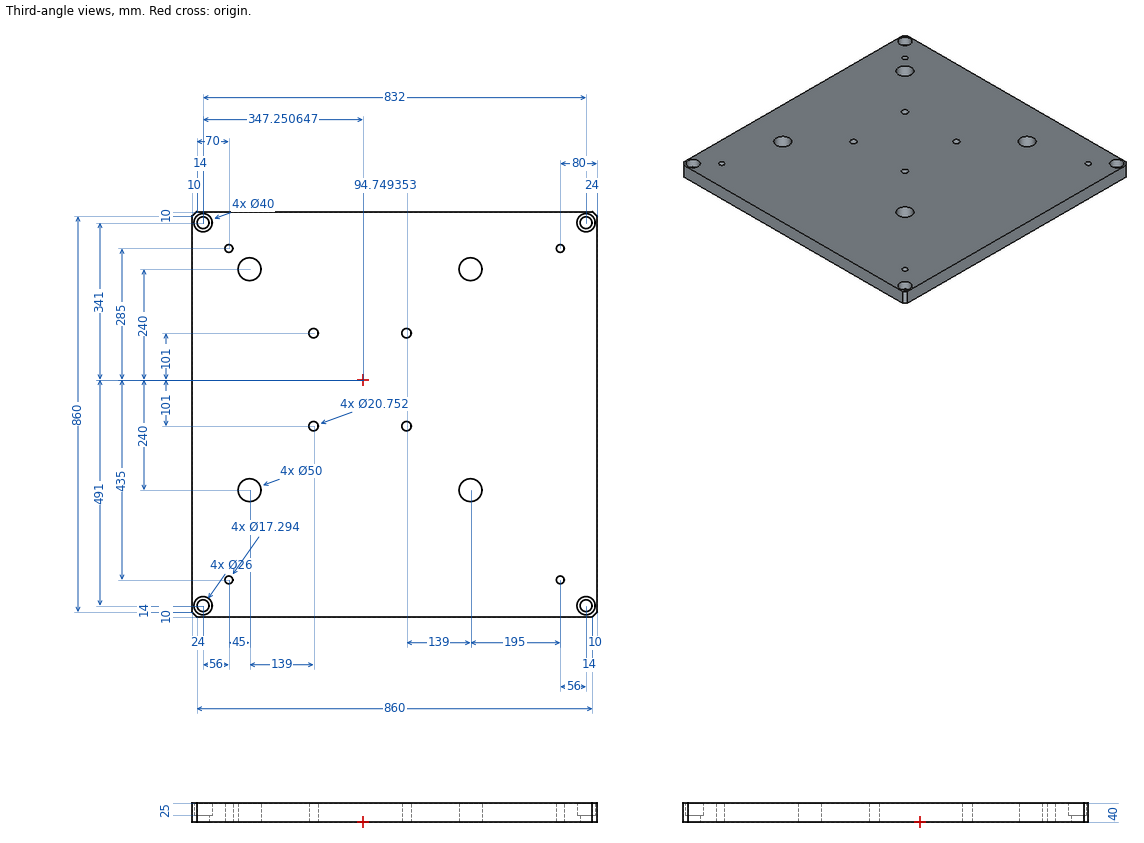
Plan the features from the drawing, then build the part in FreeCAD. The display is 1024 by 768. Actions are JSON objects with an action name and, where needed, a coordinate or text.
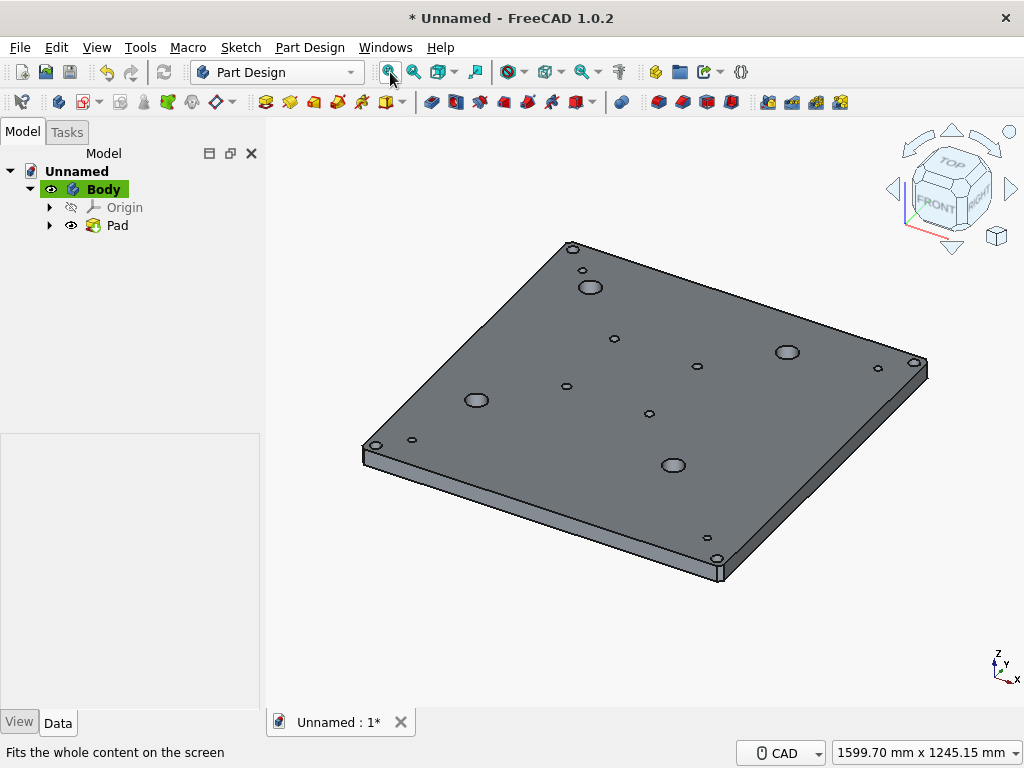
{"action": "left_click", "coordinate": [778, 408]}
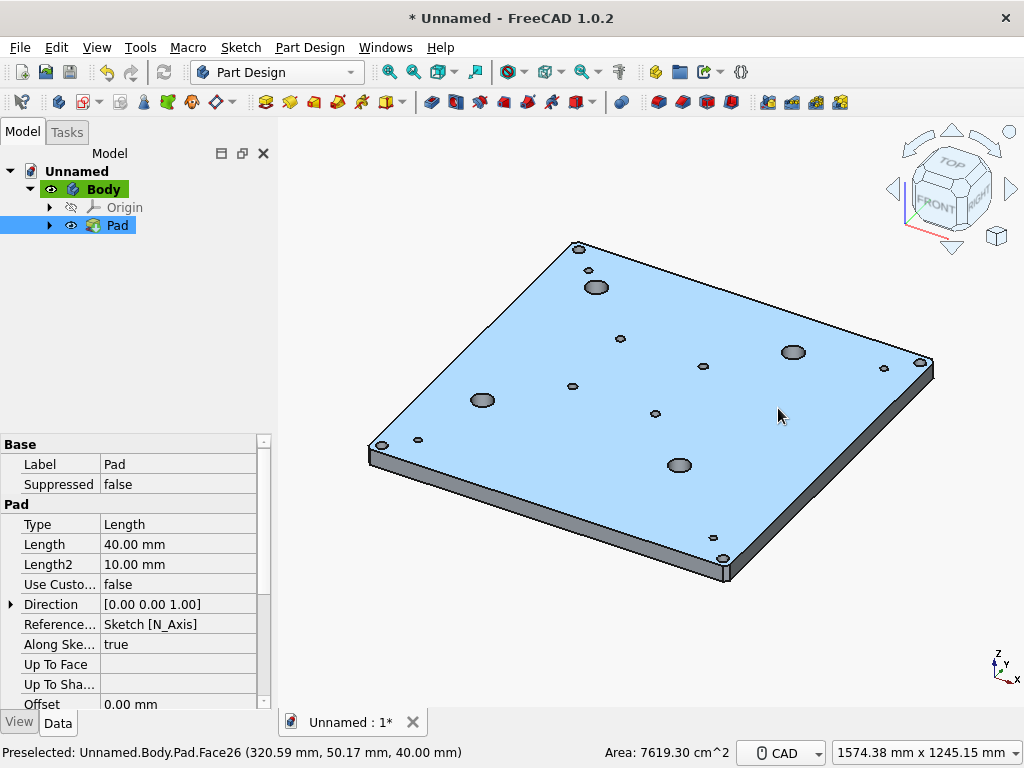
{"action": "left_click", "coordinate": [84, 102]}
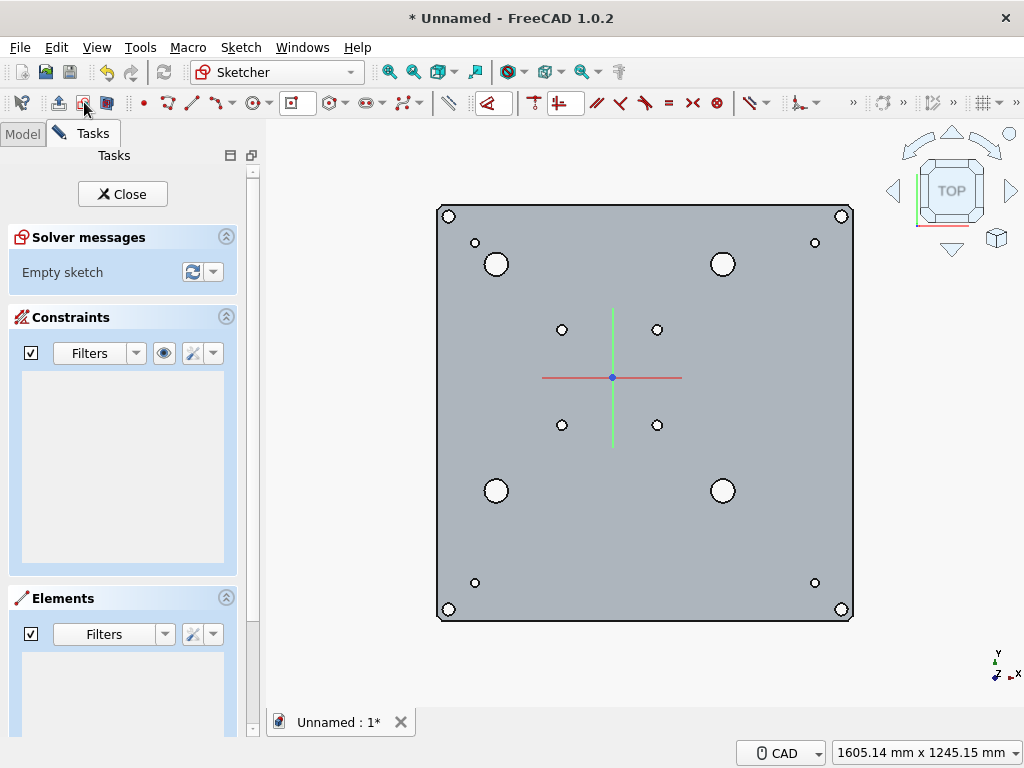
{"action": "scroll", "coordinate": [294, 413], "scroll_direction": "down", "scroll_amount": 1}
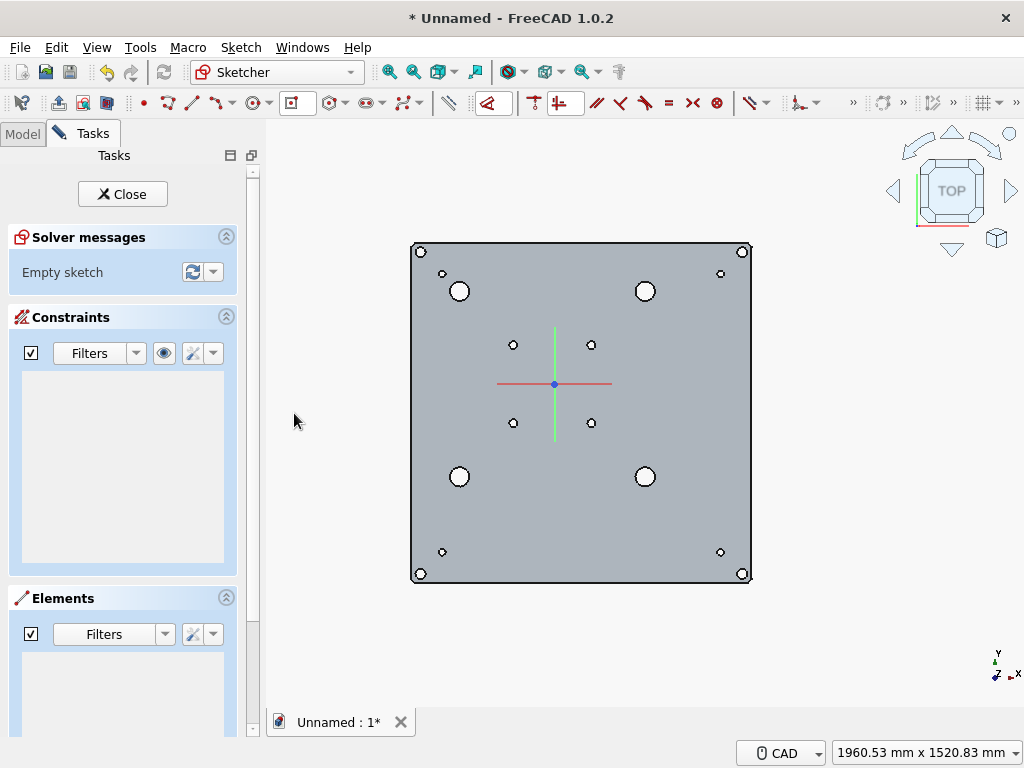
{"action": "left_click", "coordinate": [254, 104]}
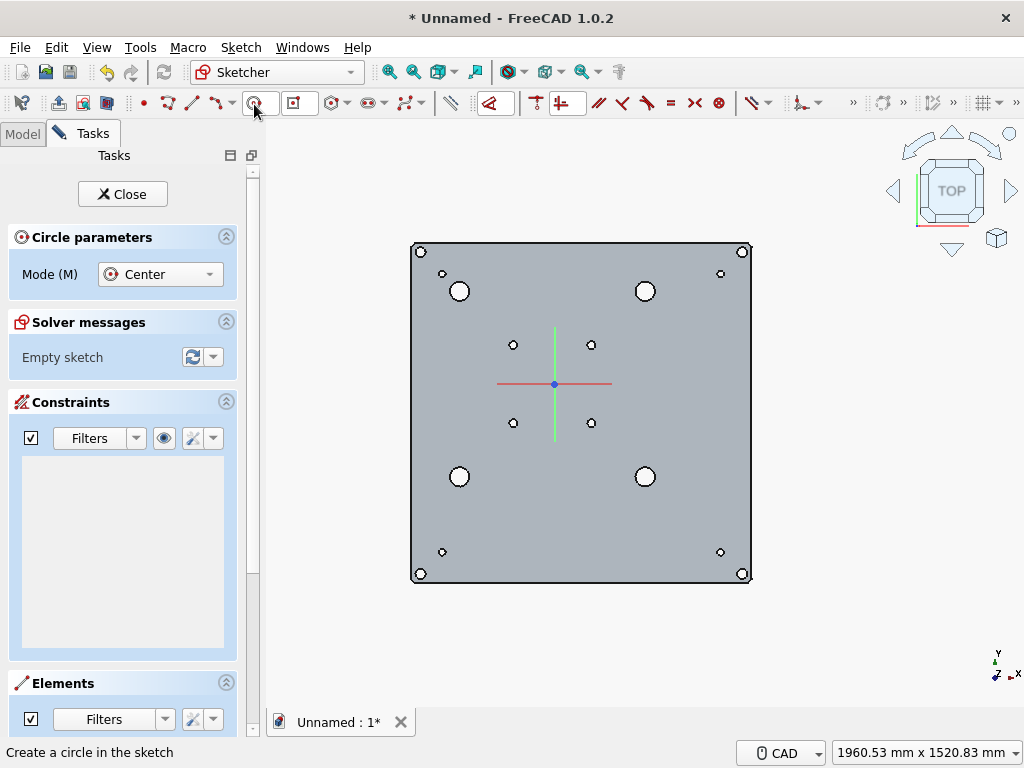
{"action": "scroll", "coordinate": [421, 252], "scroll_direction": "up", "scroll_amount": 6}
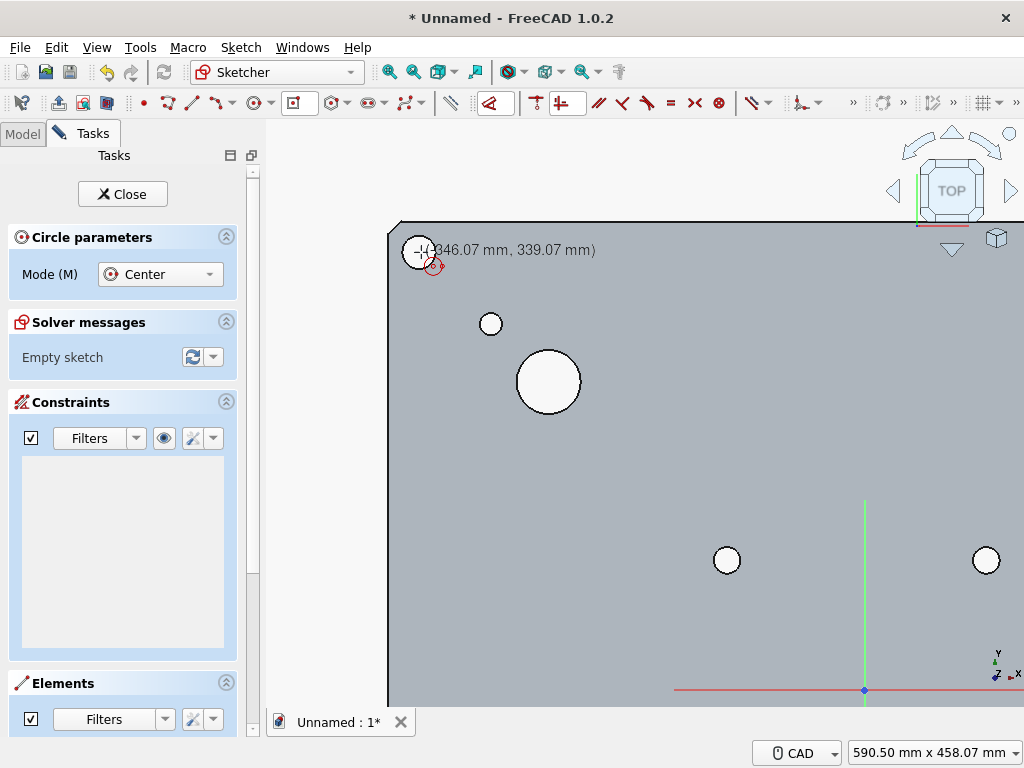
{"action": "left_click", "coordinate": [419, 252]}
{"action": "left_click", "coordinate": [437, 234]}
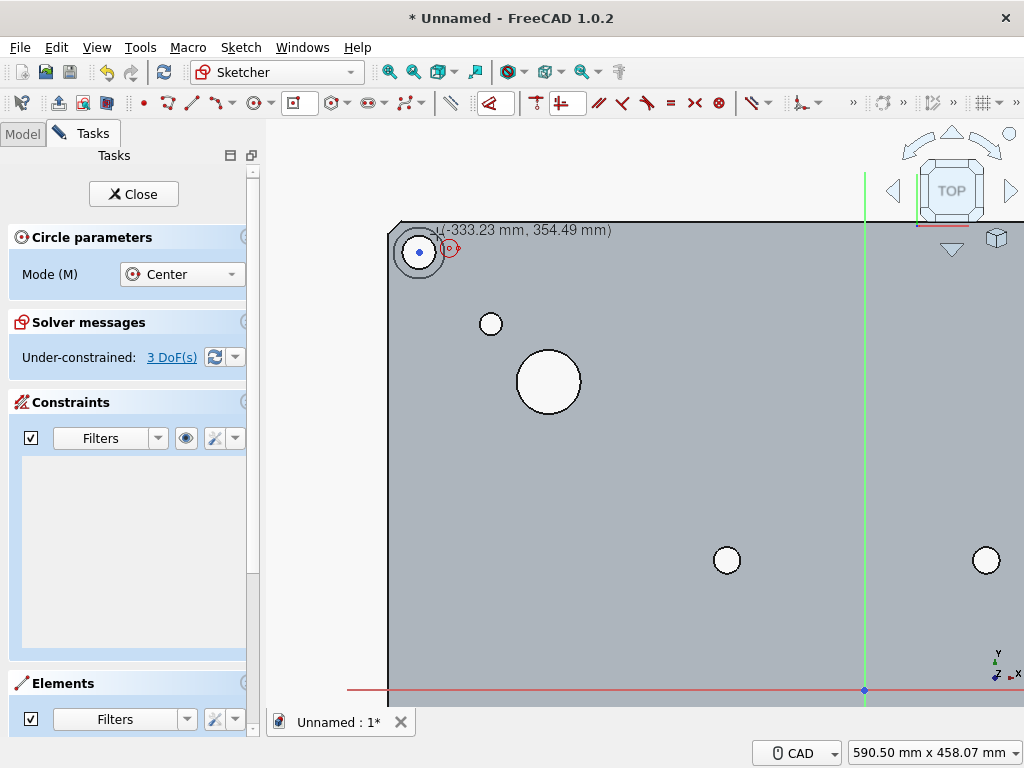
{"action": "scroll", "coordinate": [357, 196], "scroll_direction": "down", "scroll_amount": 5}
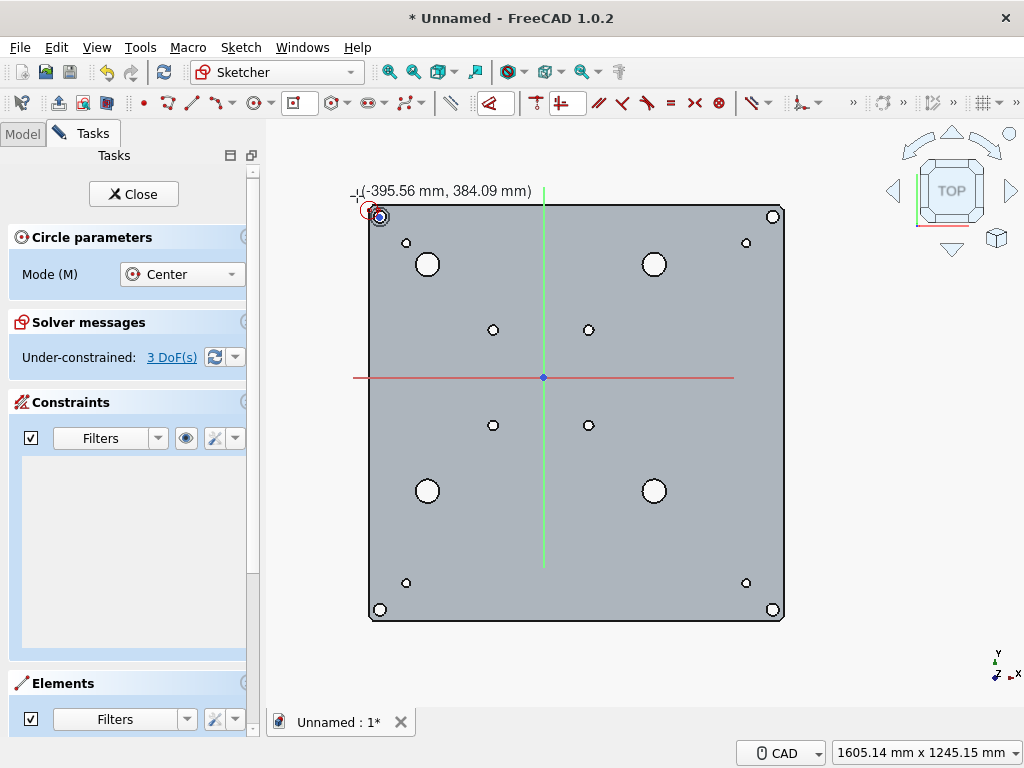
{"action": "scroll", "coordinate": [773, 217], "scroll_direction": "up", "scroll_amount": 5}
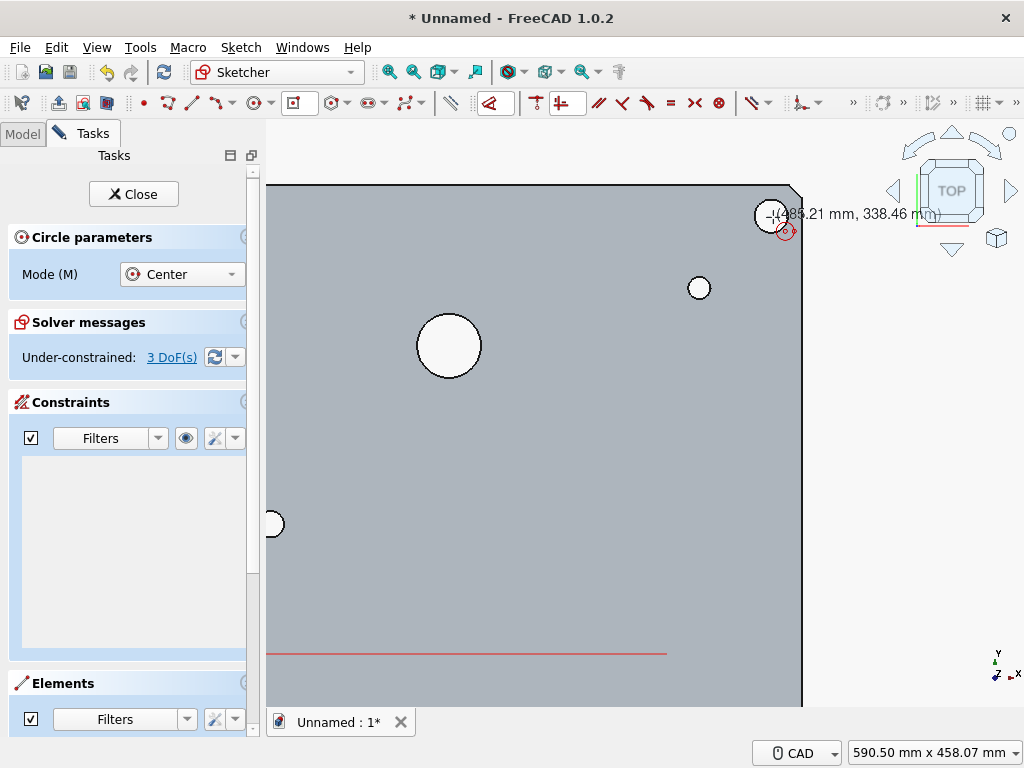
{"action": "left_click", "coordinate": [771, 216]}
{"action": "left_click", "coordinate": [789, 198]}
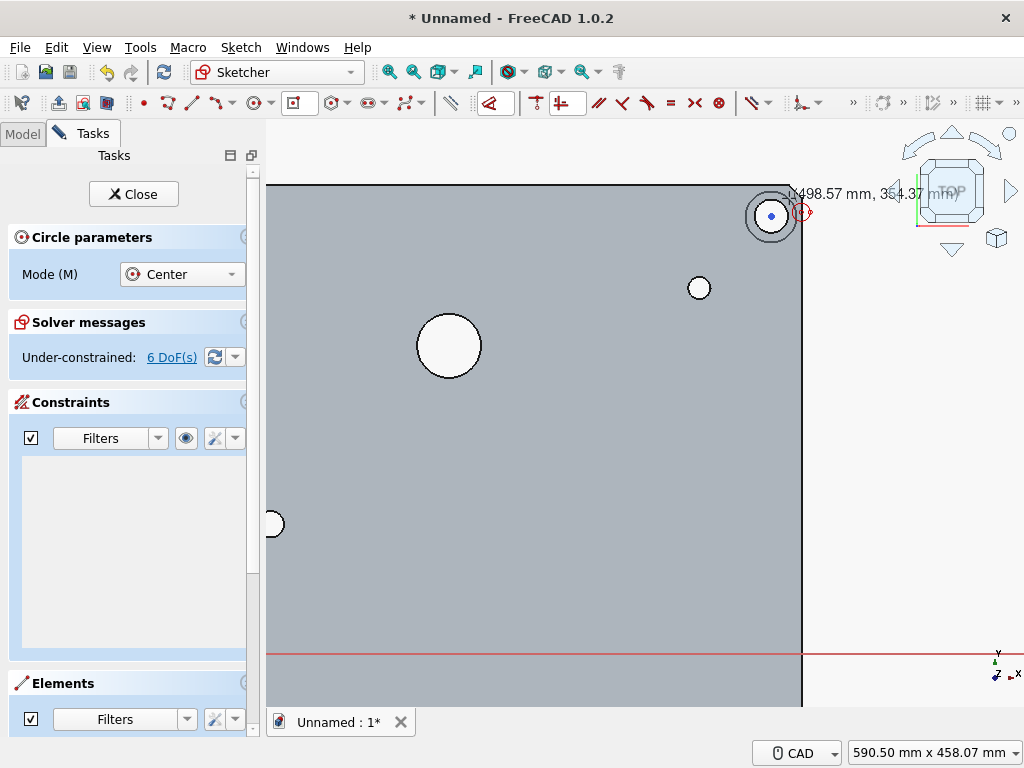
{"action": "scroll", "coordinate": [774, 217], "scroll_direction": "down", "scroll_amount": 5}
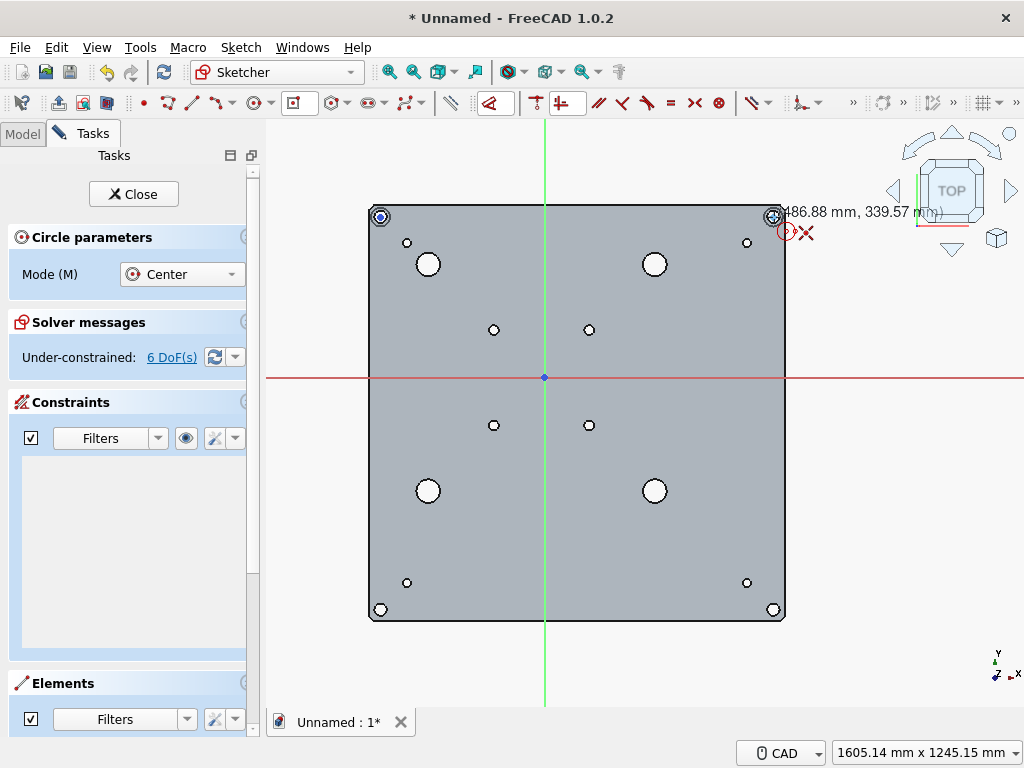
{"action": "scroll", "coordinate": [773, 610], "scroll_direction": "up", "scroll_amount": 5}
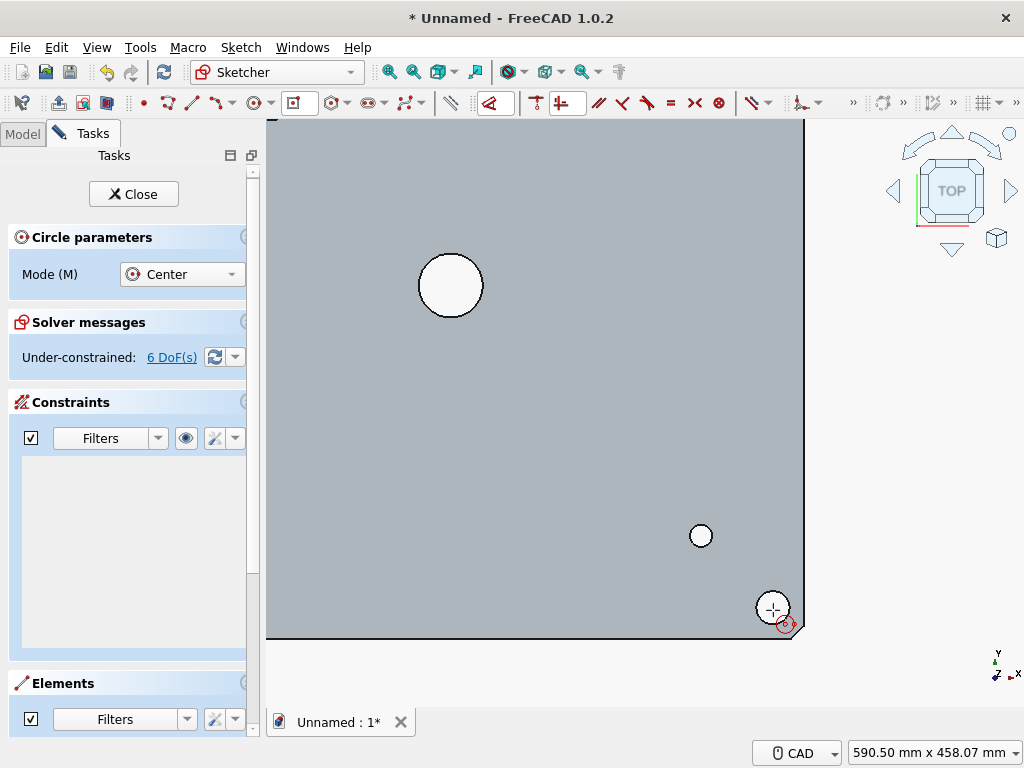
{"action": "left_click", "coordinate": [773, 608]}
{"action": "left_click", "coordinate": [791, 590]}